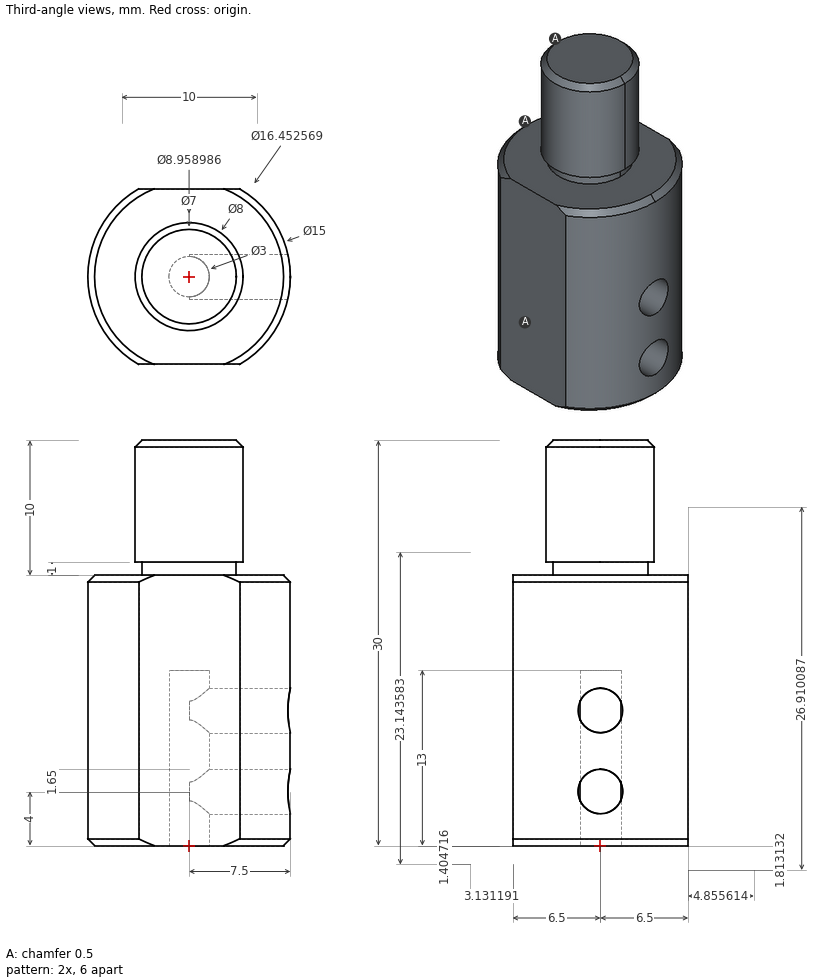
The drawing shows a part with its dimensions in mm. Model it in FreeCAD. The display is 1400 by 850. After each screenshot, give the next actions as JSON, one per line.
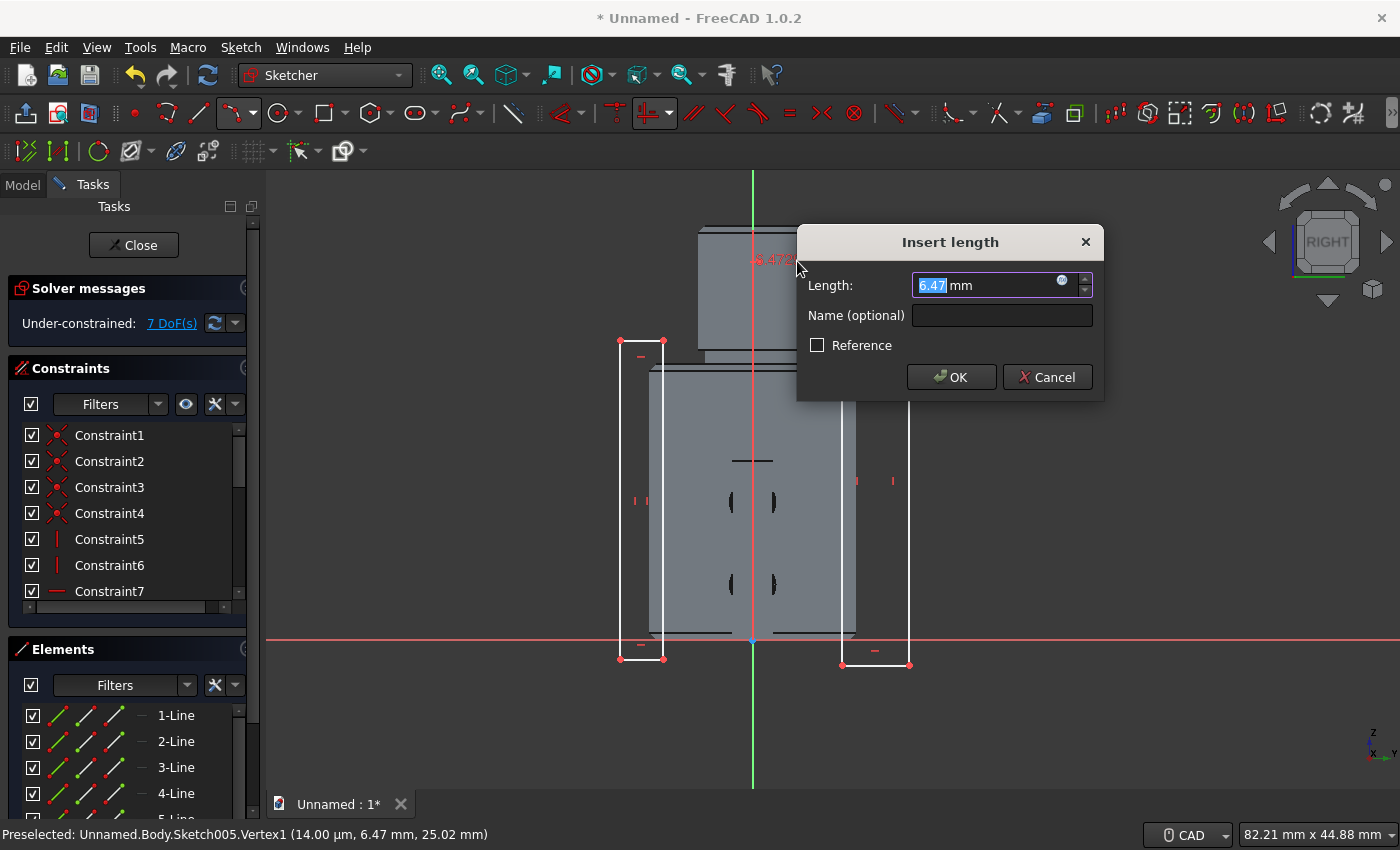
{"action": "type", "text": "6.5"}
{"action": "key", "text": "Return"}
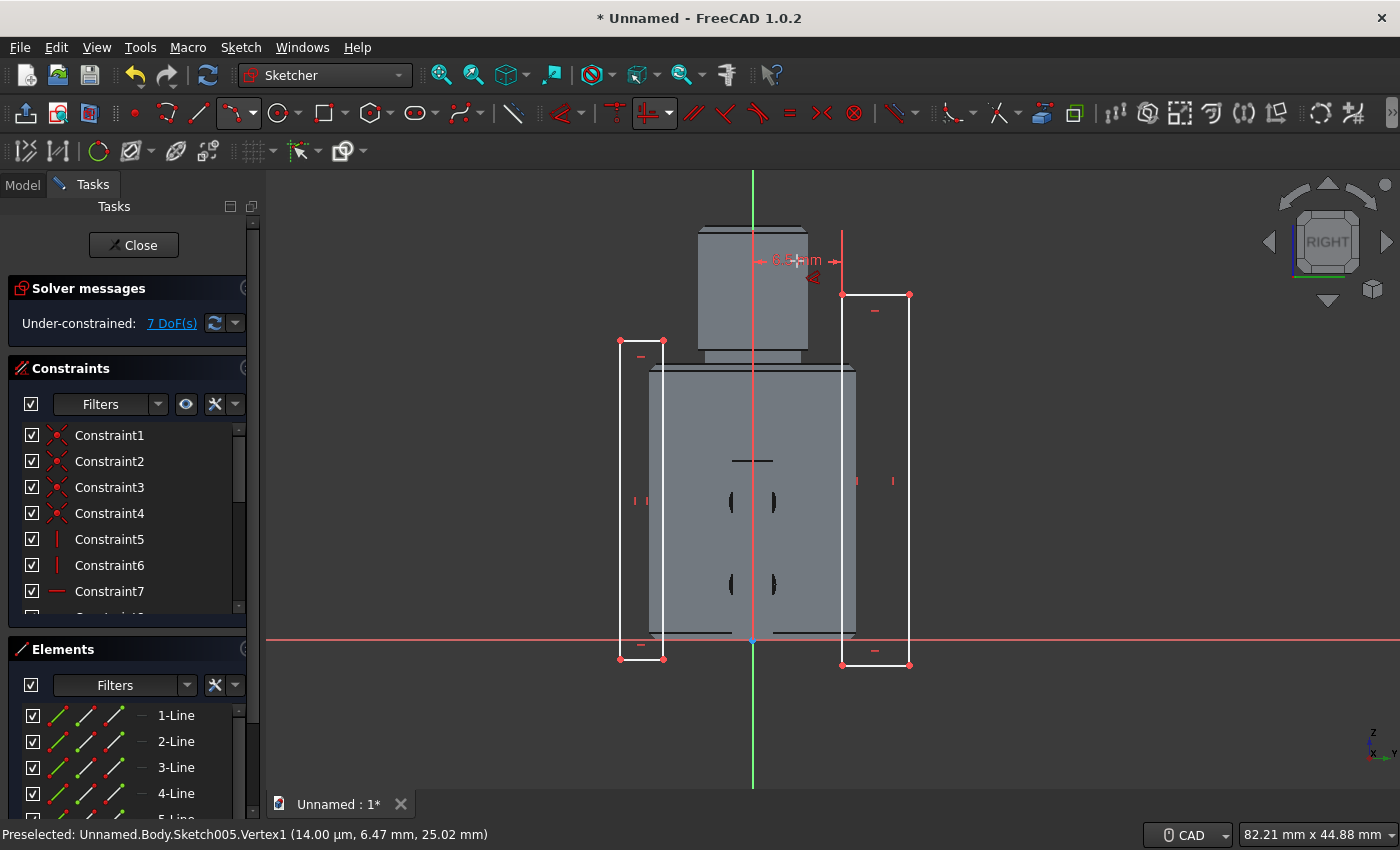
{"action": "left_click", "coordinate": [663, 660]}
{"action": "left_click", "coordinate": [708, 694]}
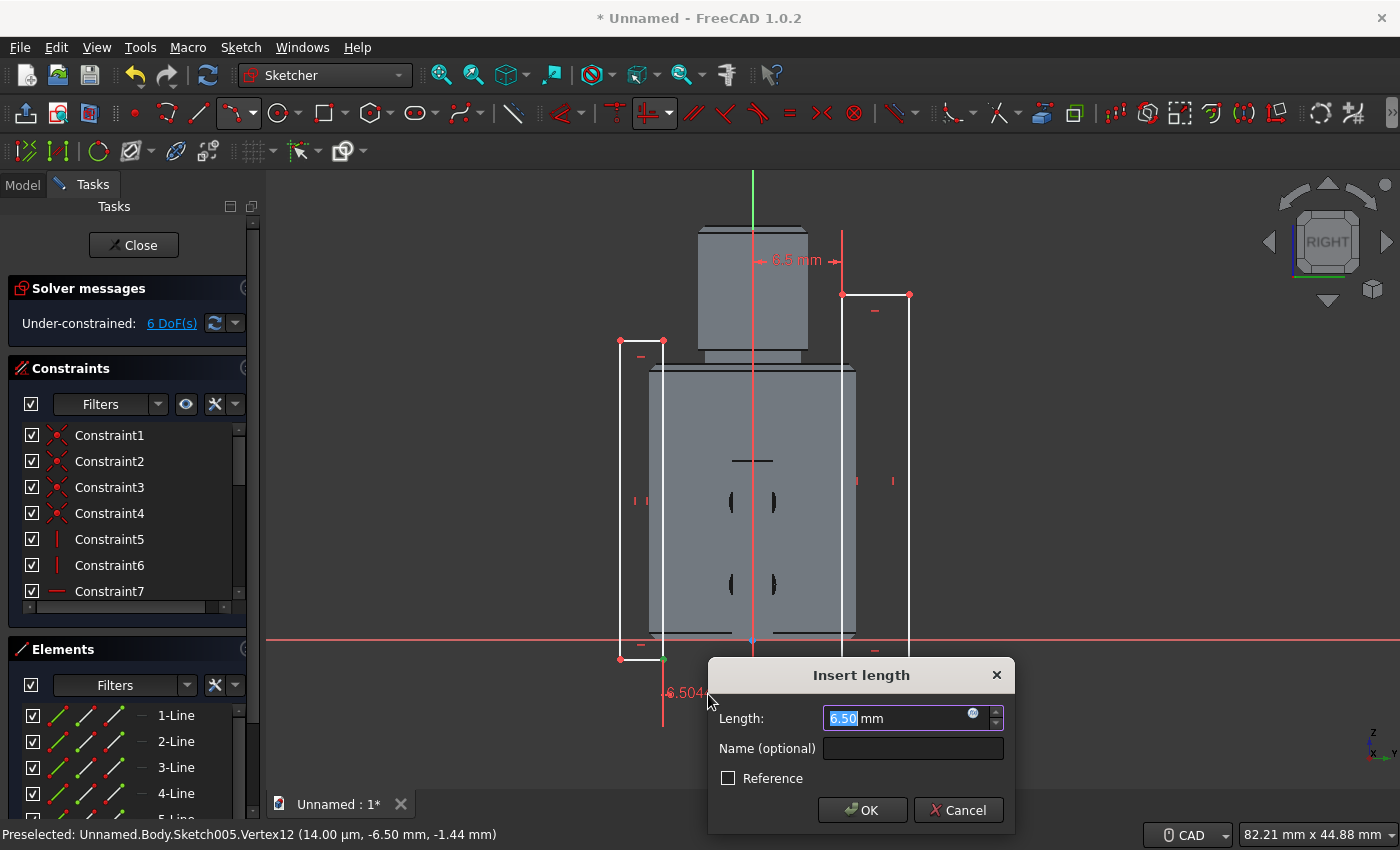
{"action": "type", "text": "6.5"}
{"action": "key", "text": "Return"}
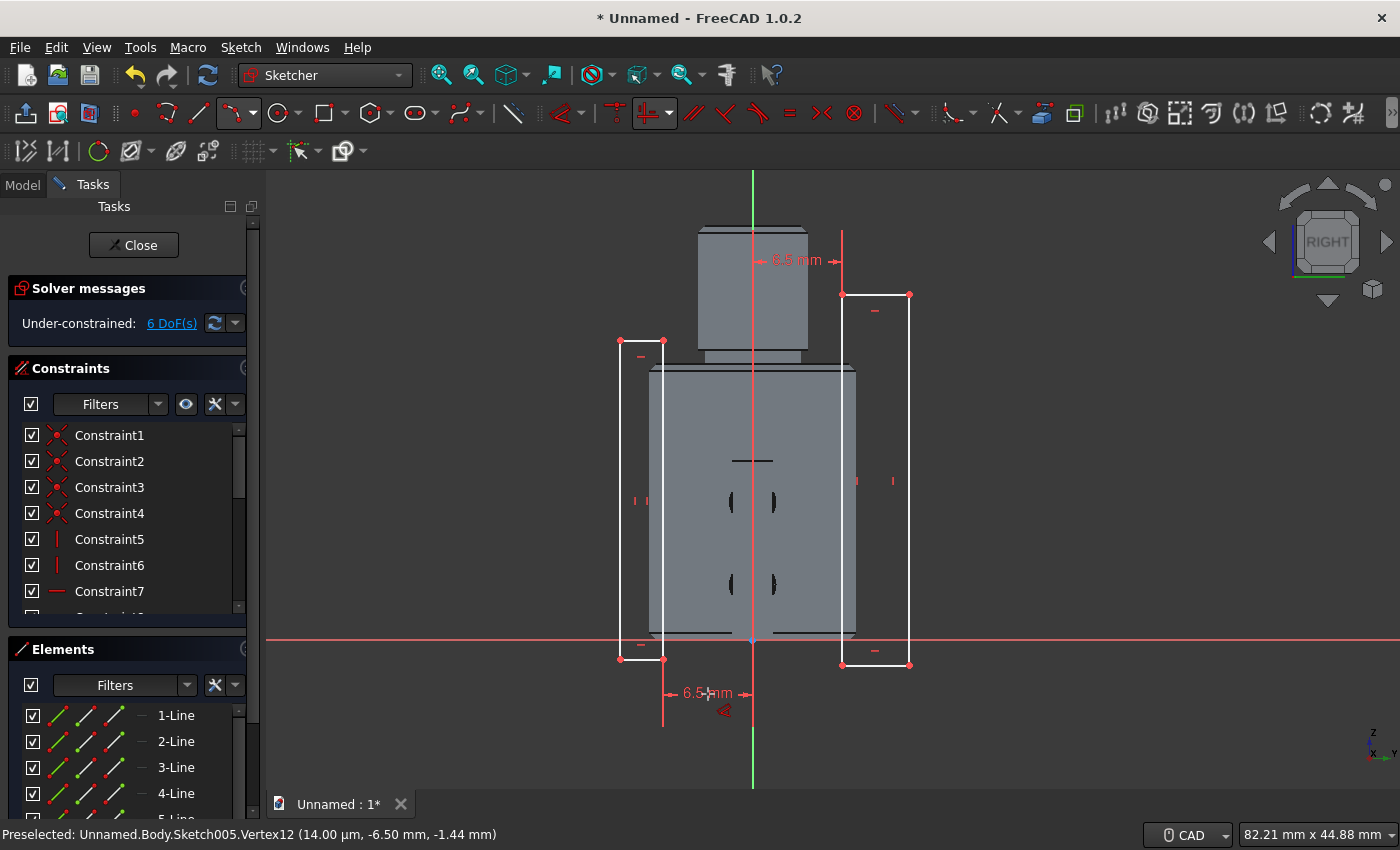
{"action": "left_click", "coordinate": [862, 666]}
{"action": "left_click", "coordinate": [876, 700]}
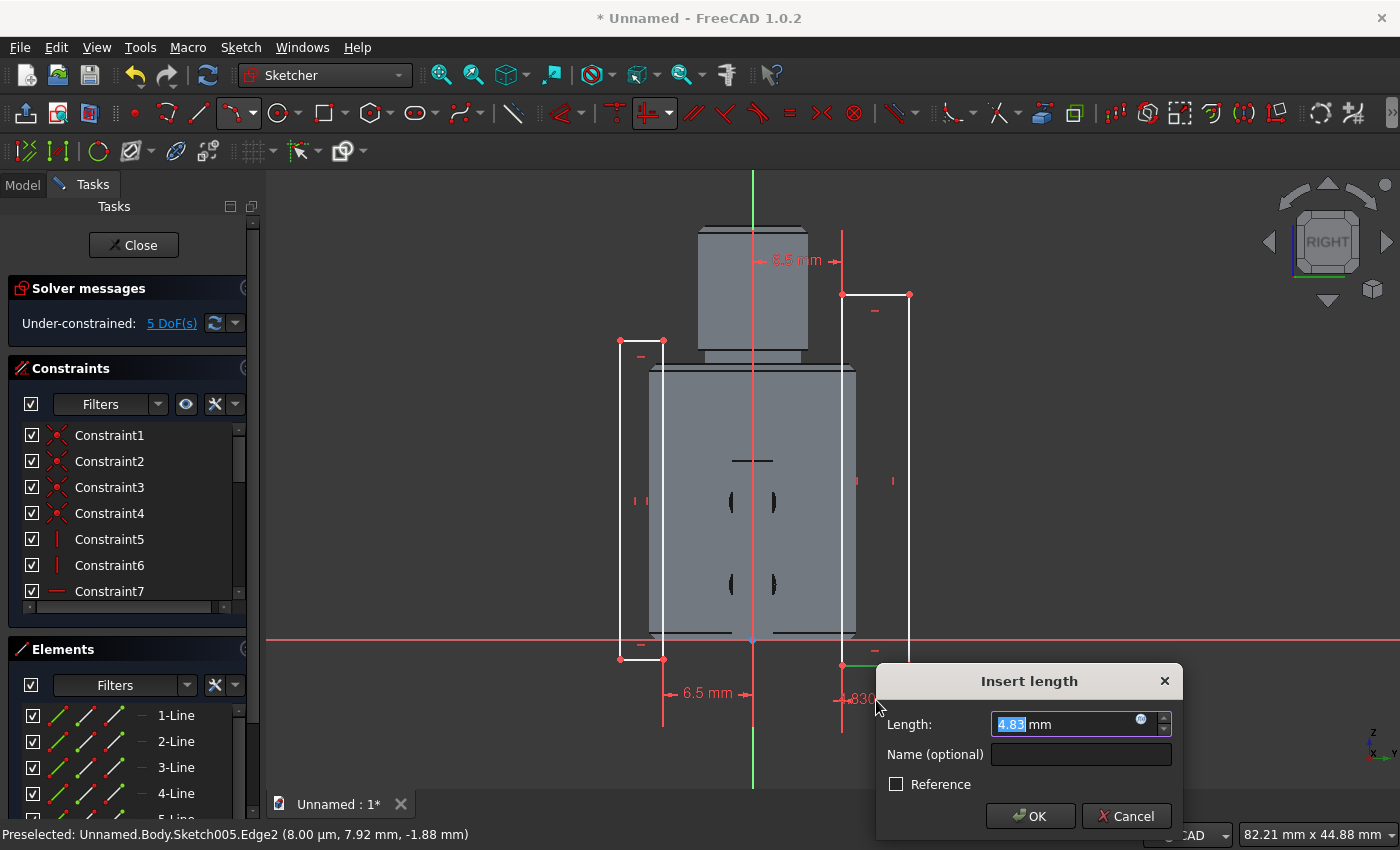
{"action": "type", "text": "4.855614"}
{"action": "key", "text": "Return"}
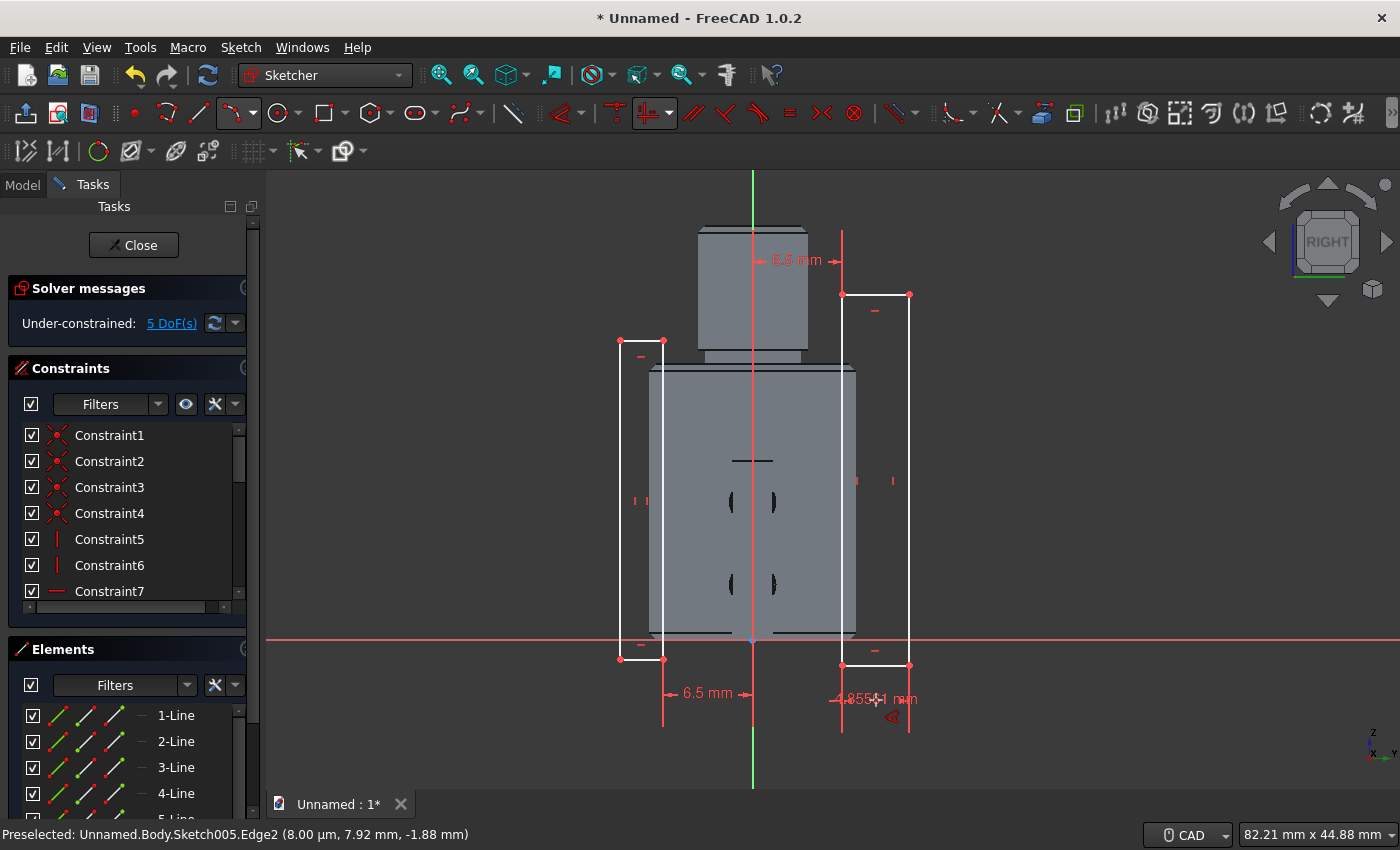
{"action": "left_click", "coordinate": [633, 660]}
{"action": "left_click", "coordinate": [632, 694]}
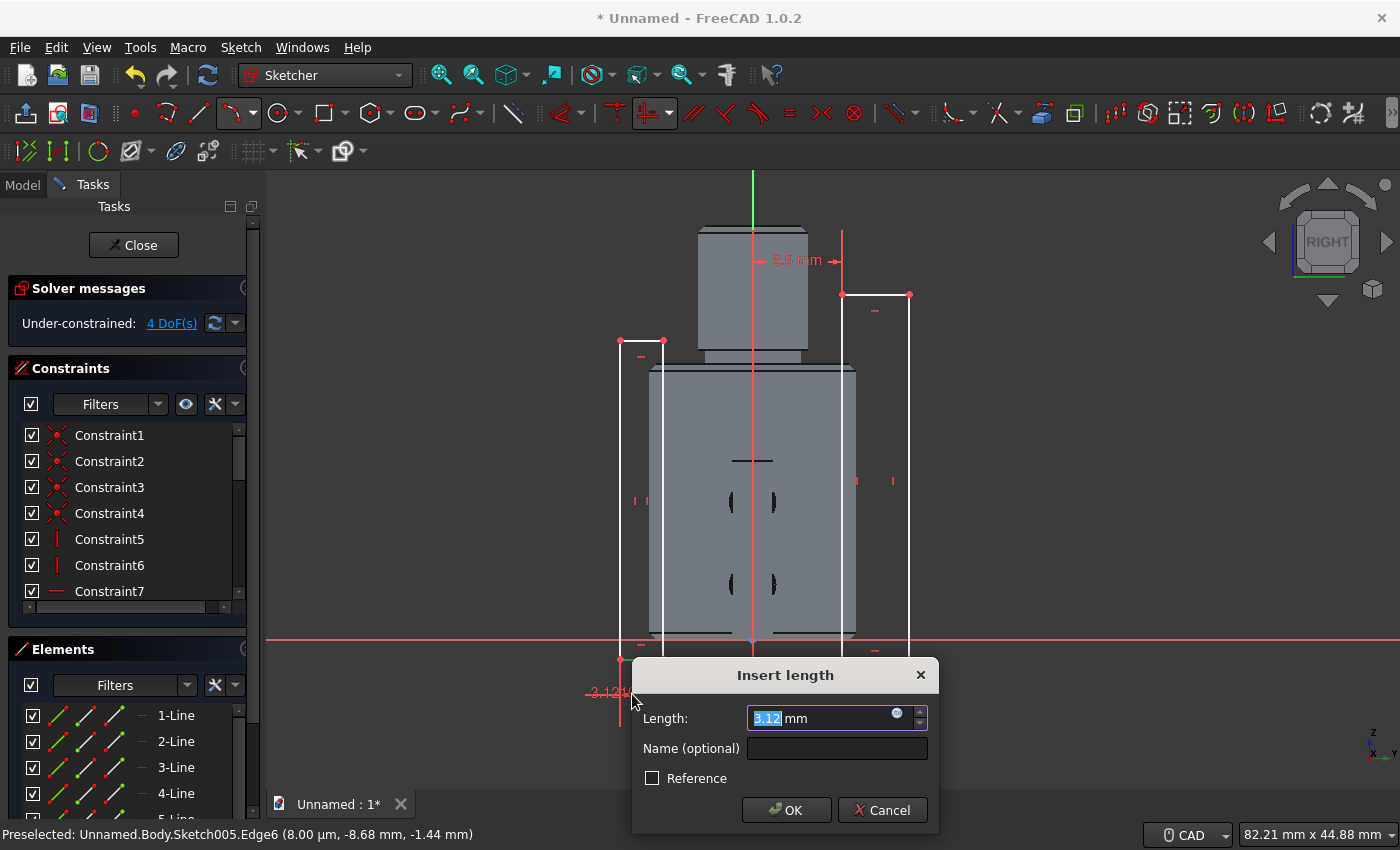
{"action": "type", "text": "3.131191"}
{"action": "key", "text": "Return"}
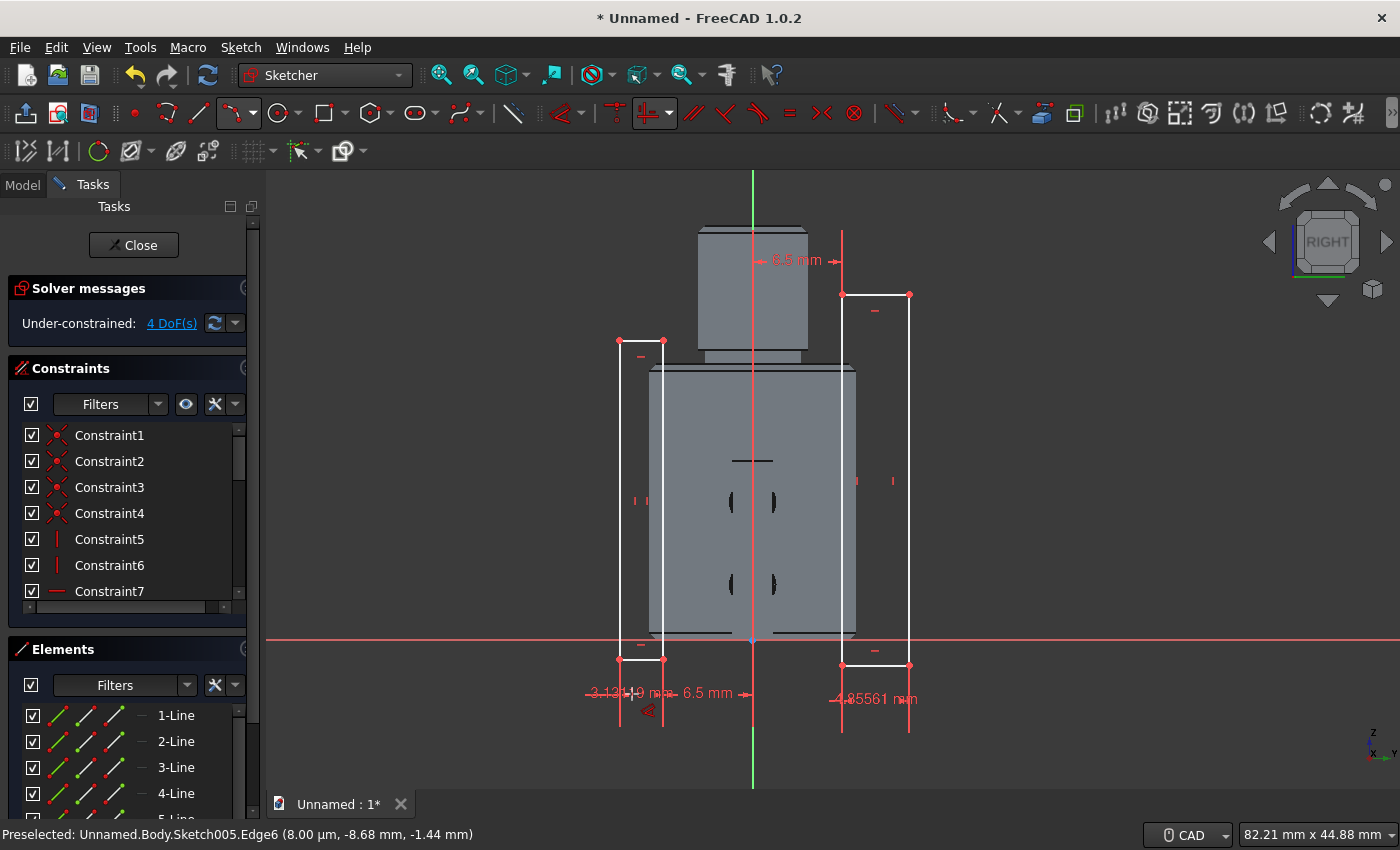
{"action": "left_click", "coordinate": [842, 406]}
{"action": "left_click", "coordinate": [876, 481]}